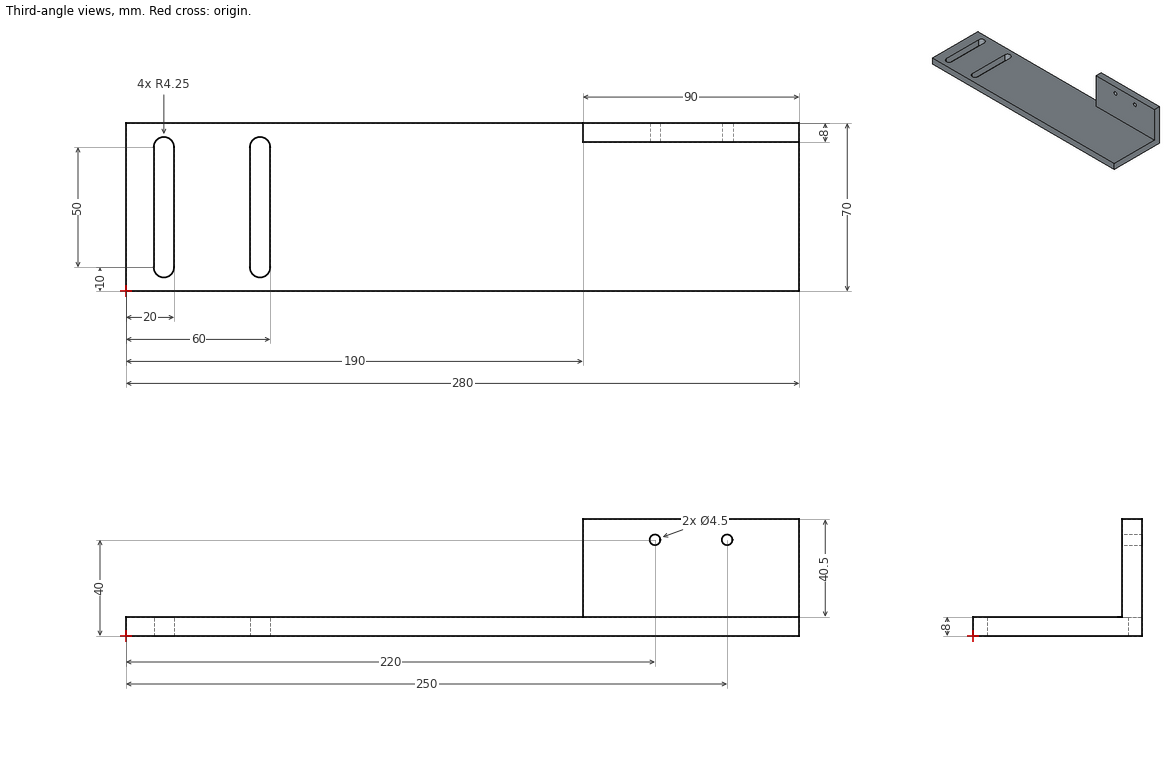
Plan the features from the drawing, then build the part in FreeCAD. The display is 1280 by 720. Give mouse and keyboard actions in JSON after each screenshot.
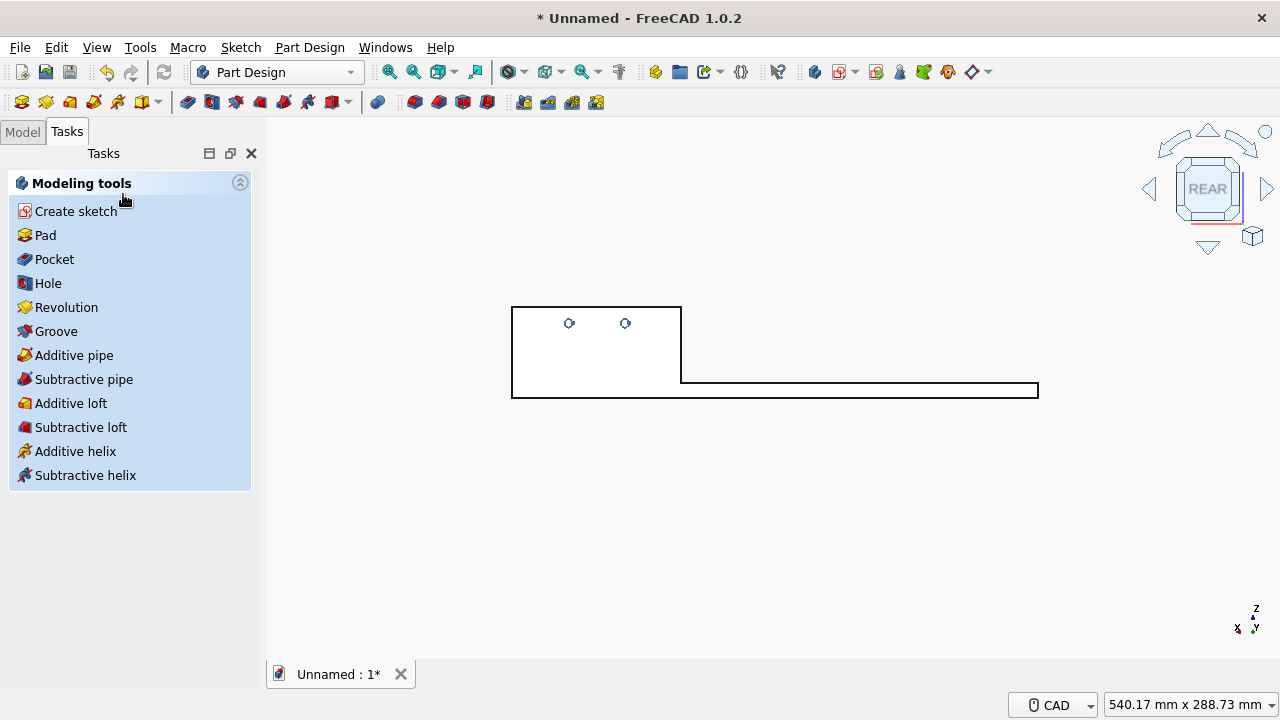
{"action": "left_click", "coordinate": [188, 102]}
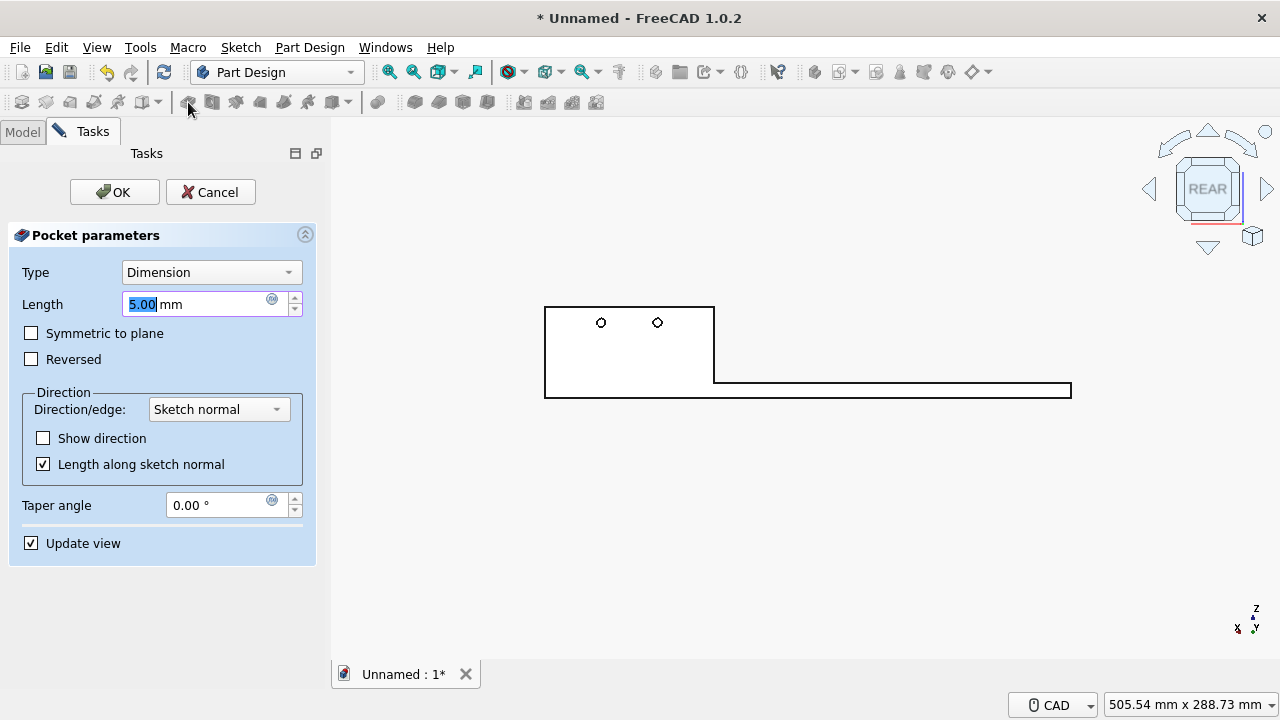
{"action": "left_click", "coordinate": [212, 272]}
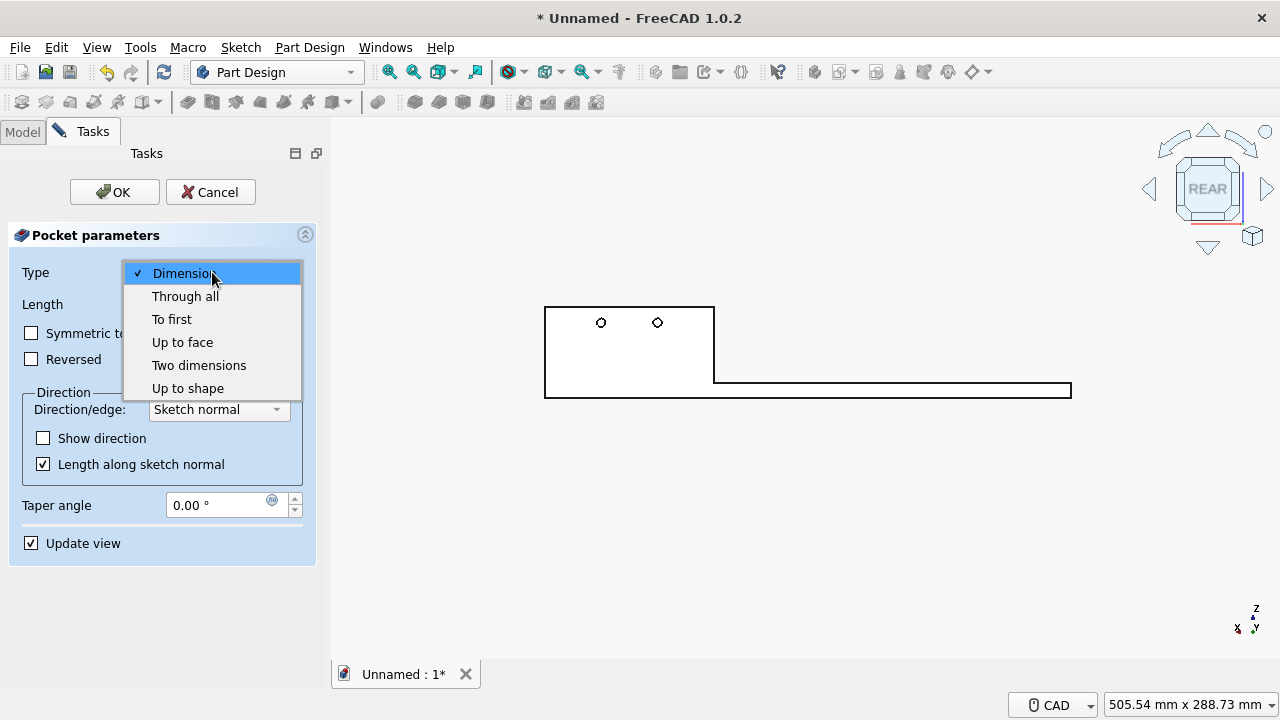
{"action": "left_click", "coordinate": [212, 296]}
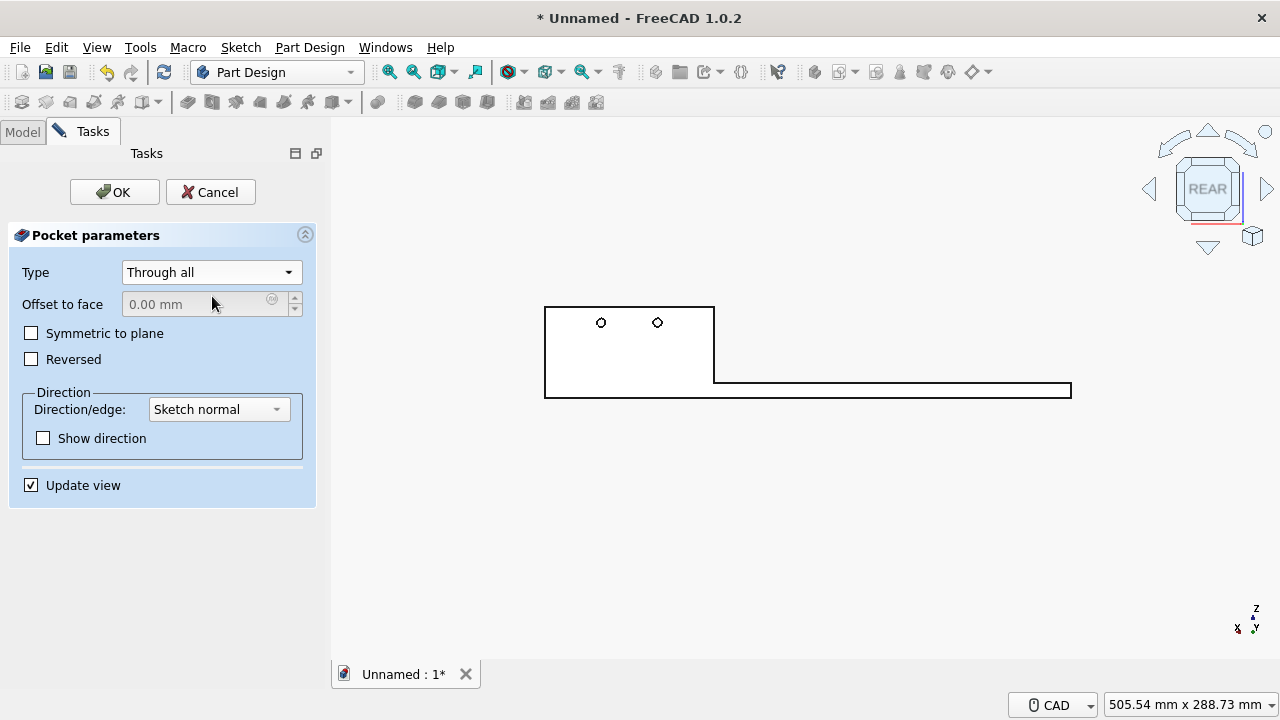
{"action": "left_click", "coordinate": [115, 192]}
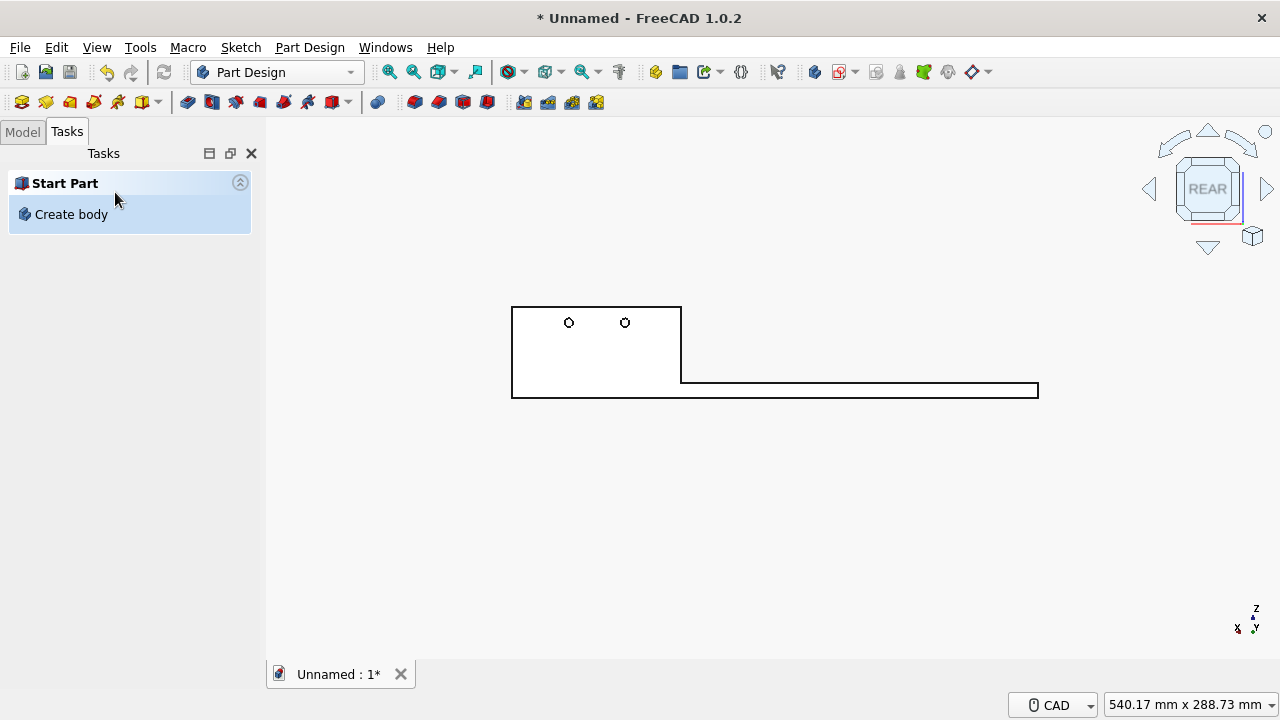
{"action": "key", "text": "0"}